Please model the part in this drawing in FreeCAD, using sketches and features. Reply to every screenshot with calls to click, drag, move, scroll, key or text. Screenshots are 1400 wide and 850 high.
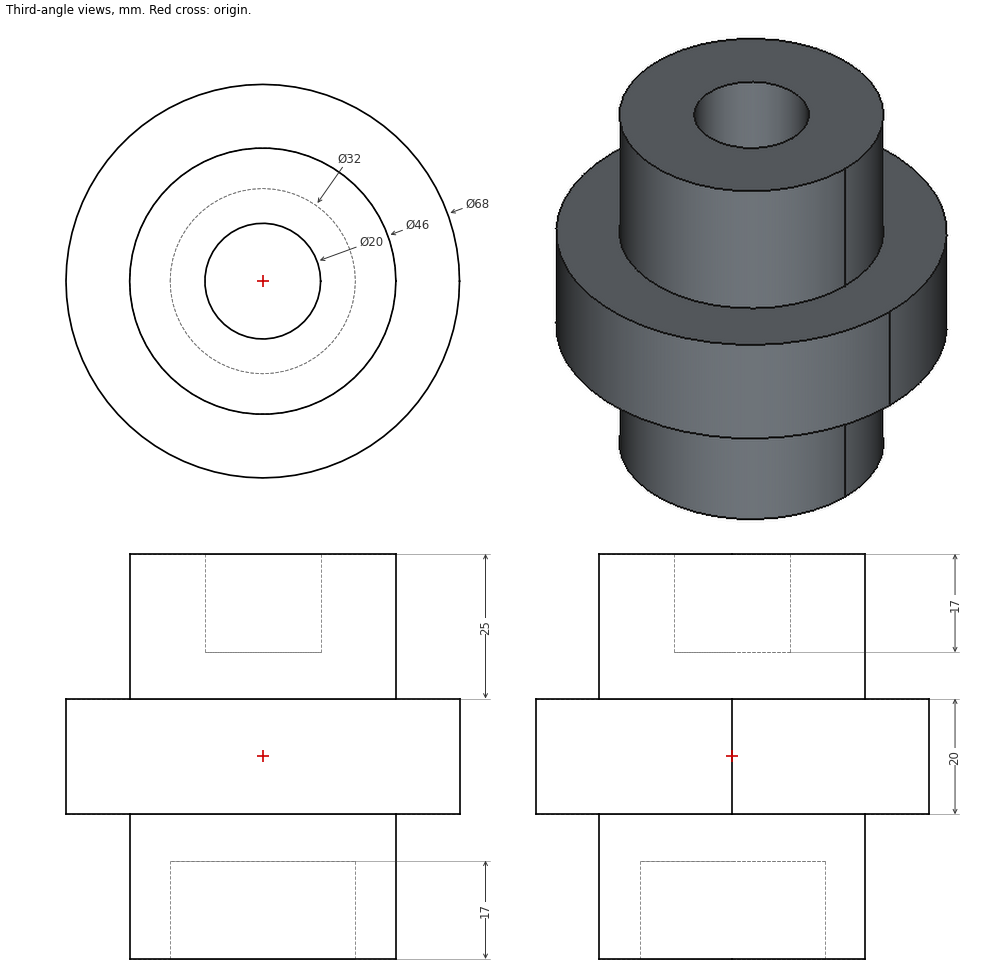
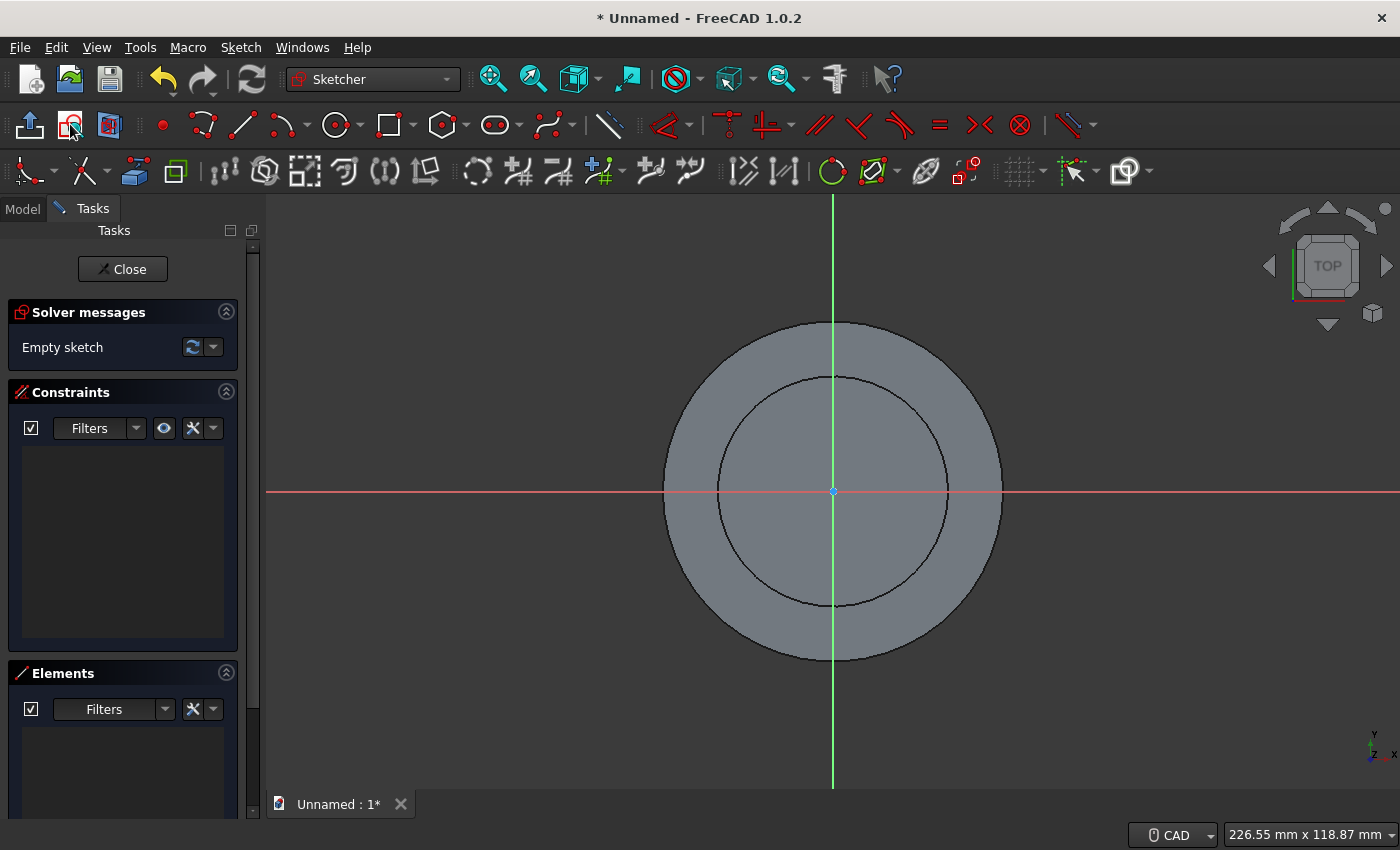
scroll(855, 492, up, 7)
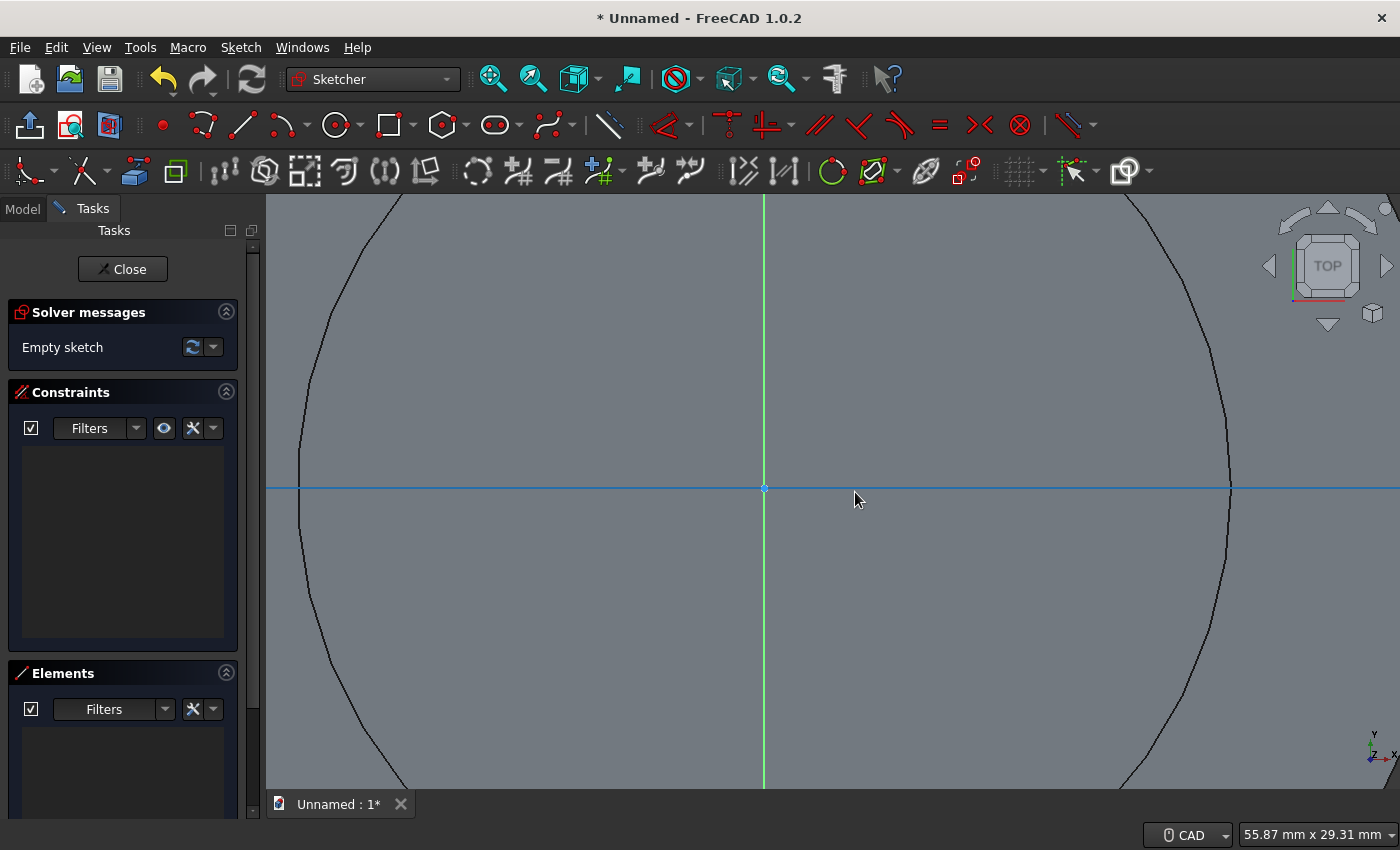
click(336, 126)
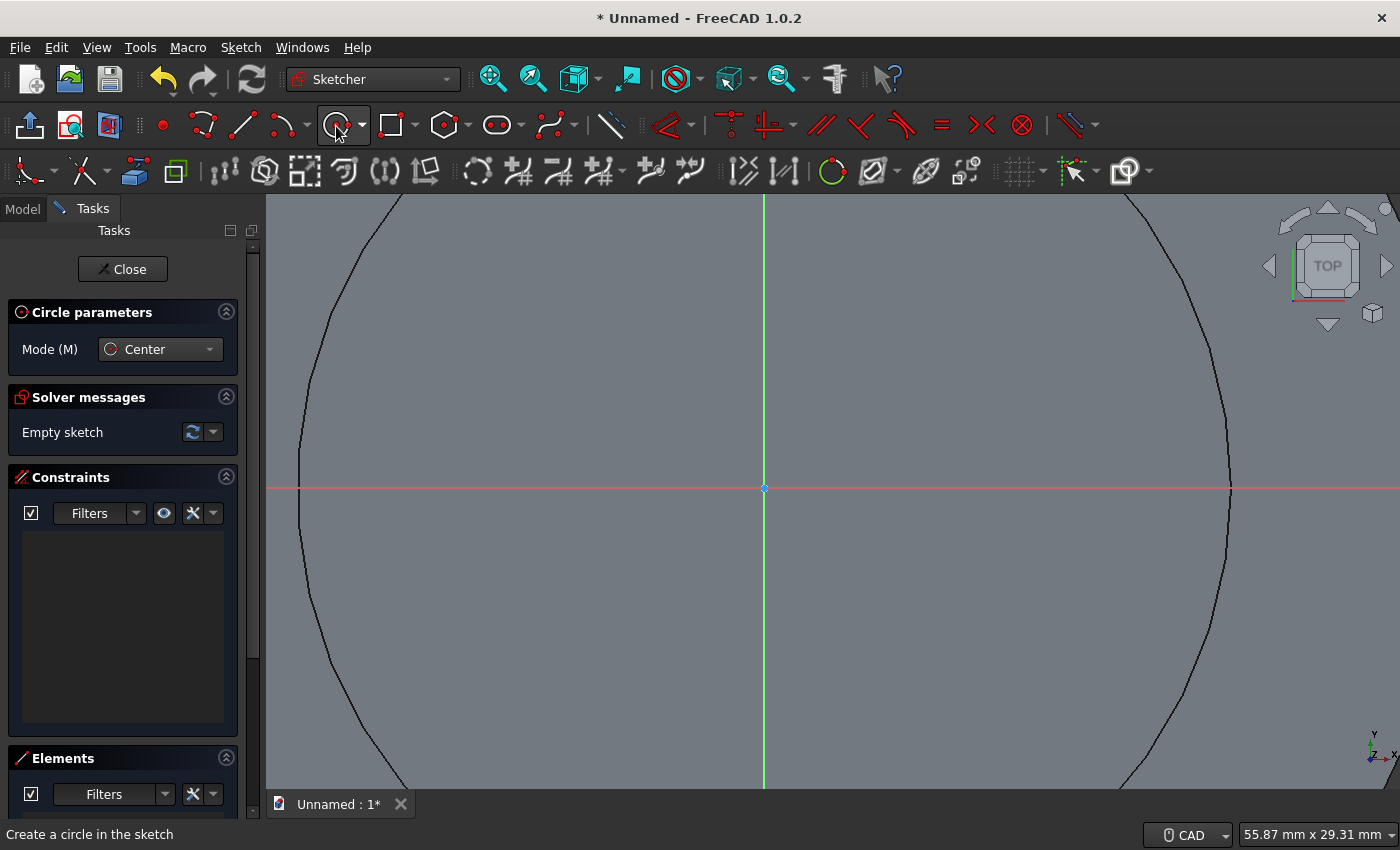
click(764, 488)
move(908, 345)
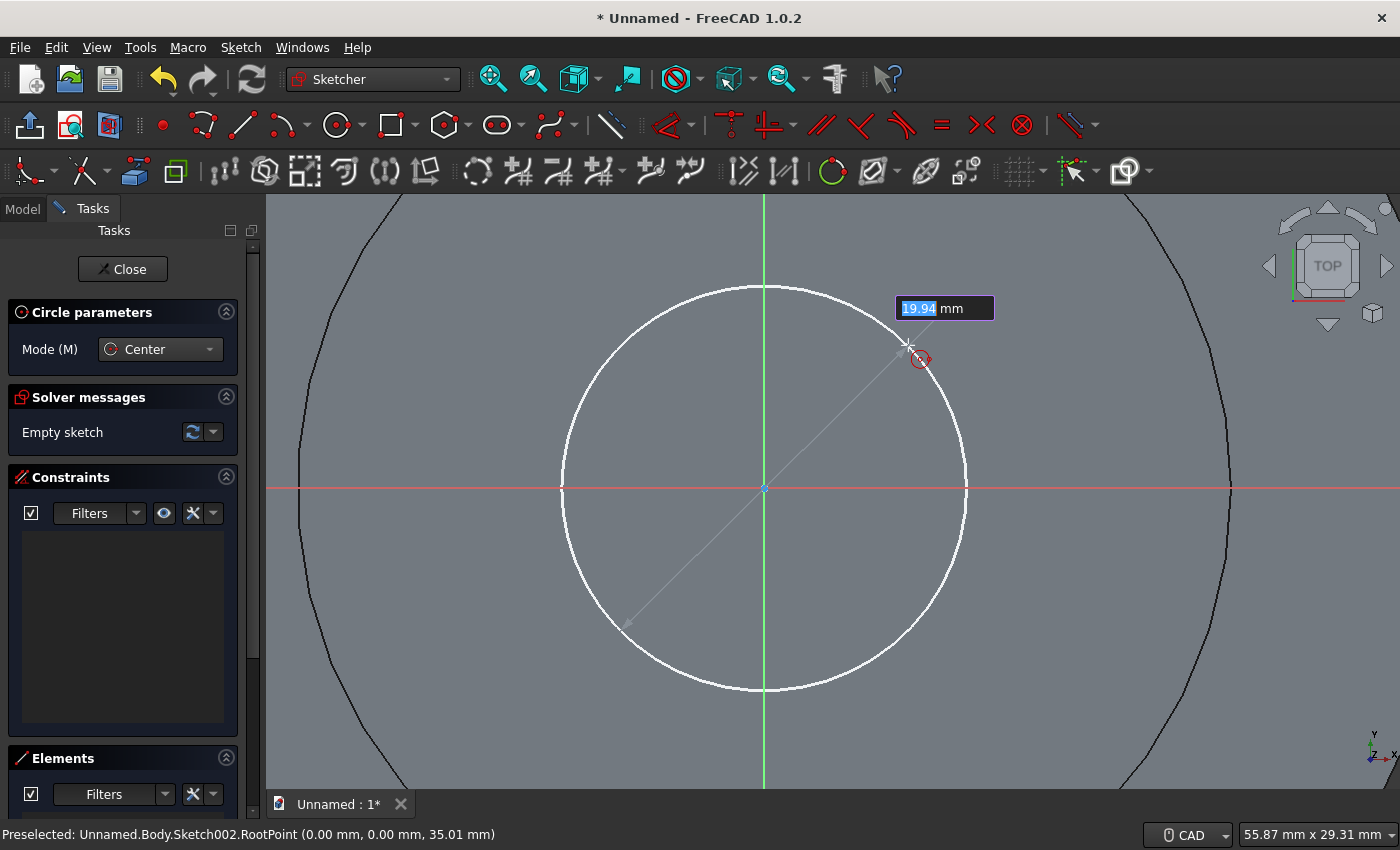
text(20)
key(Return)
key(Escape)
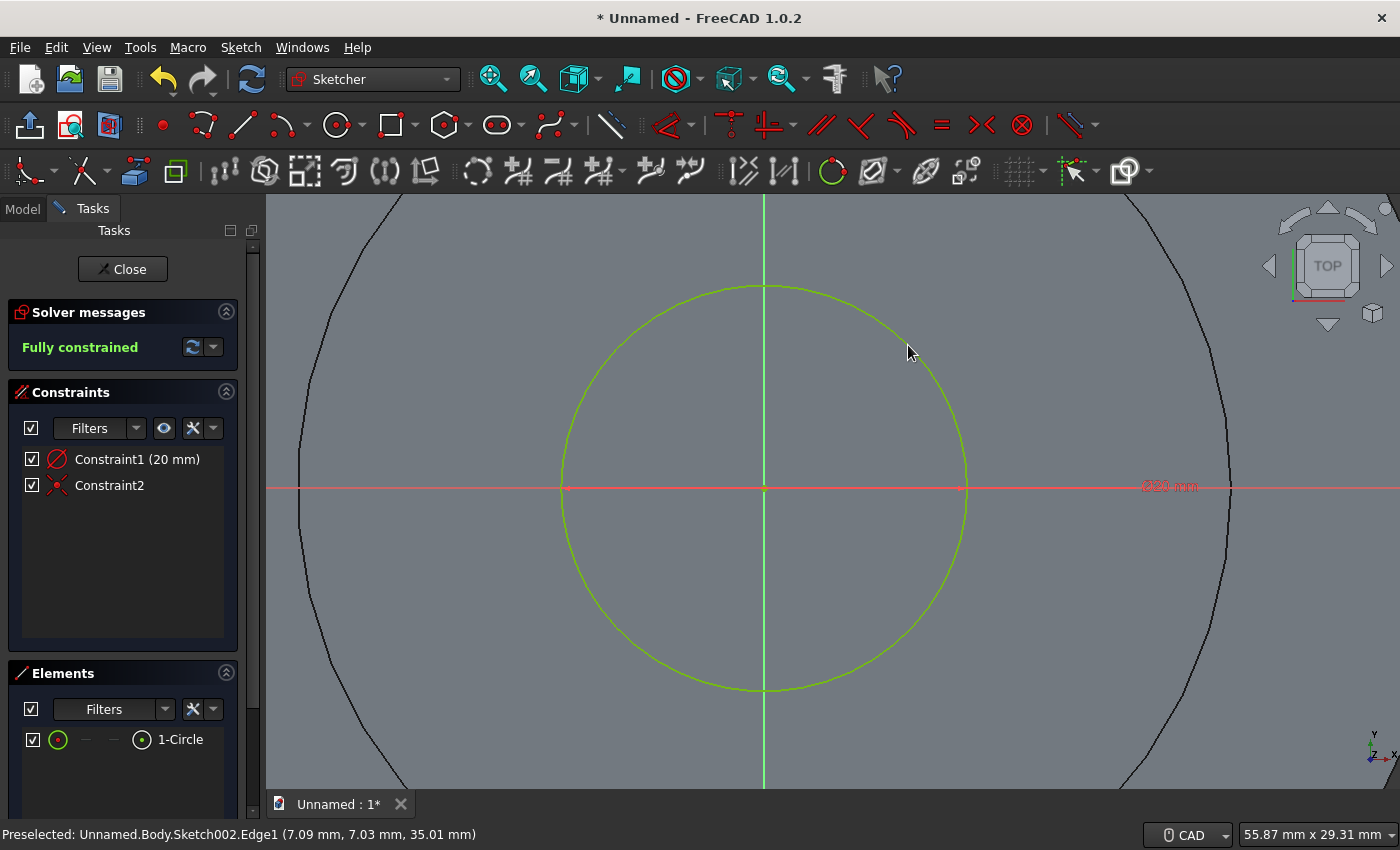
click(123, 269)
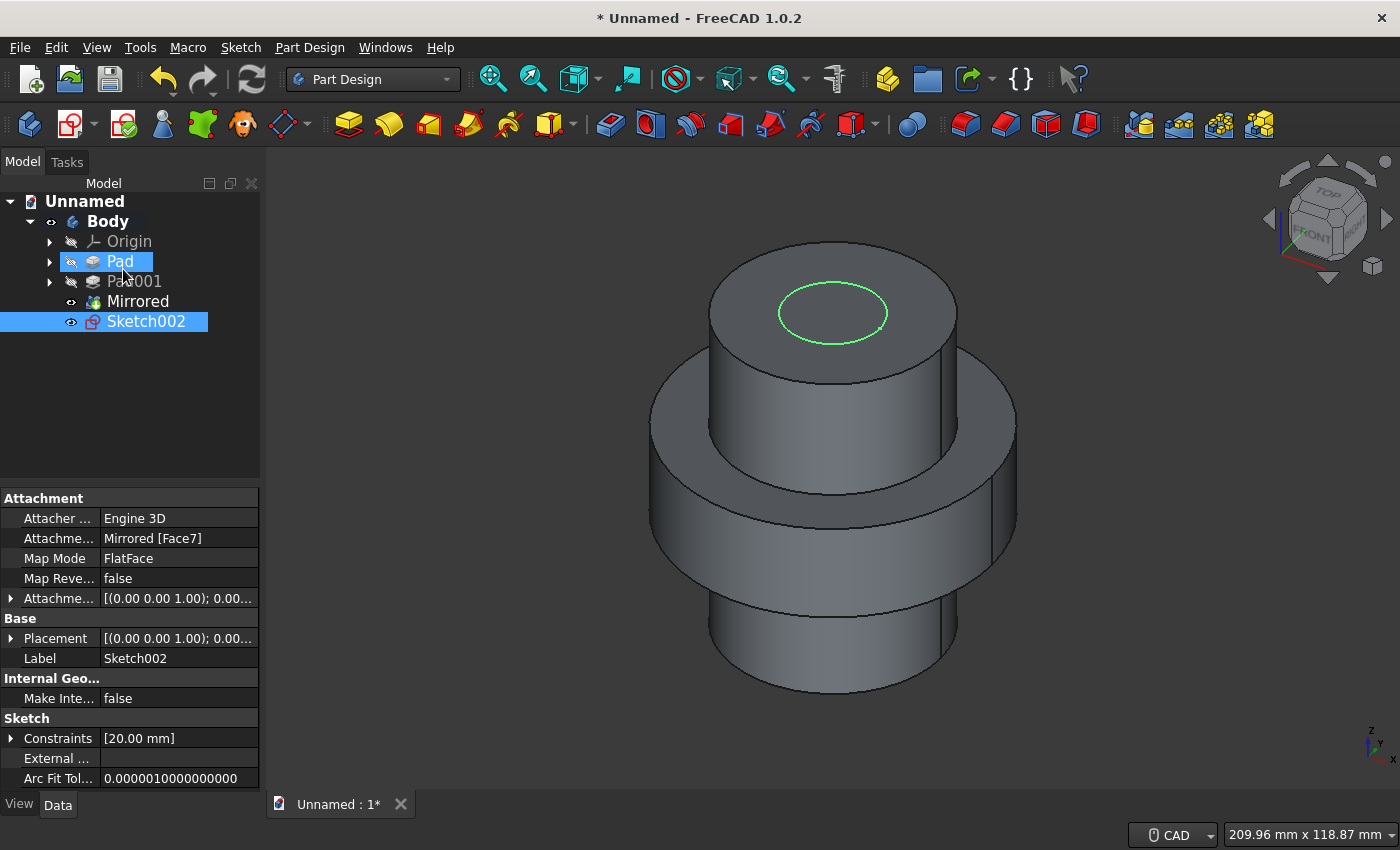
click(612, 124)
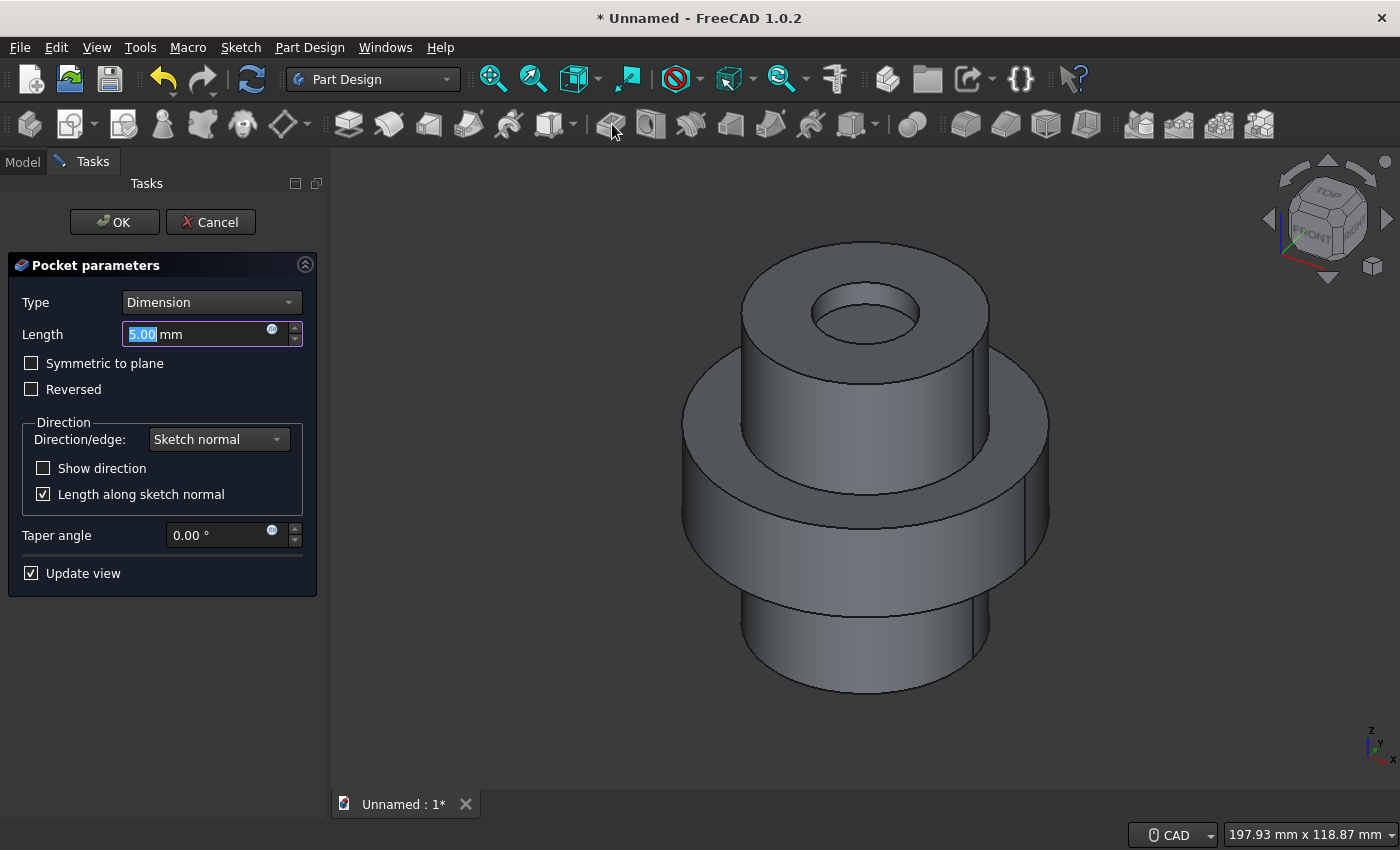
text(17)
key(Tab)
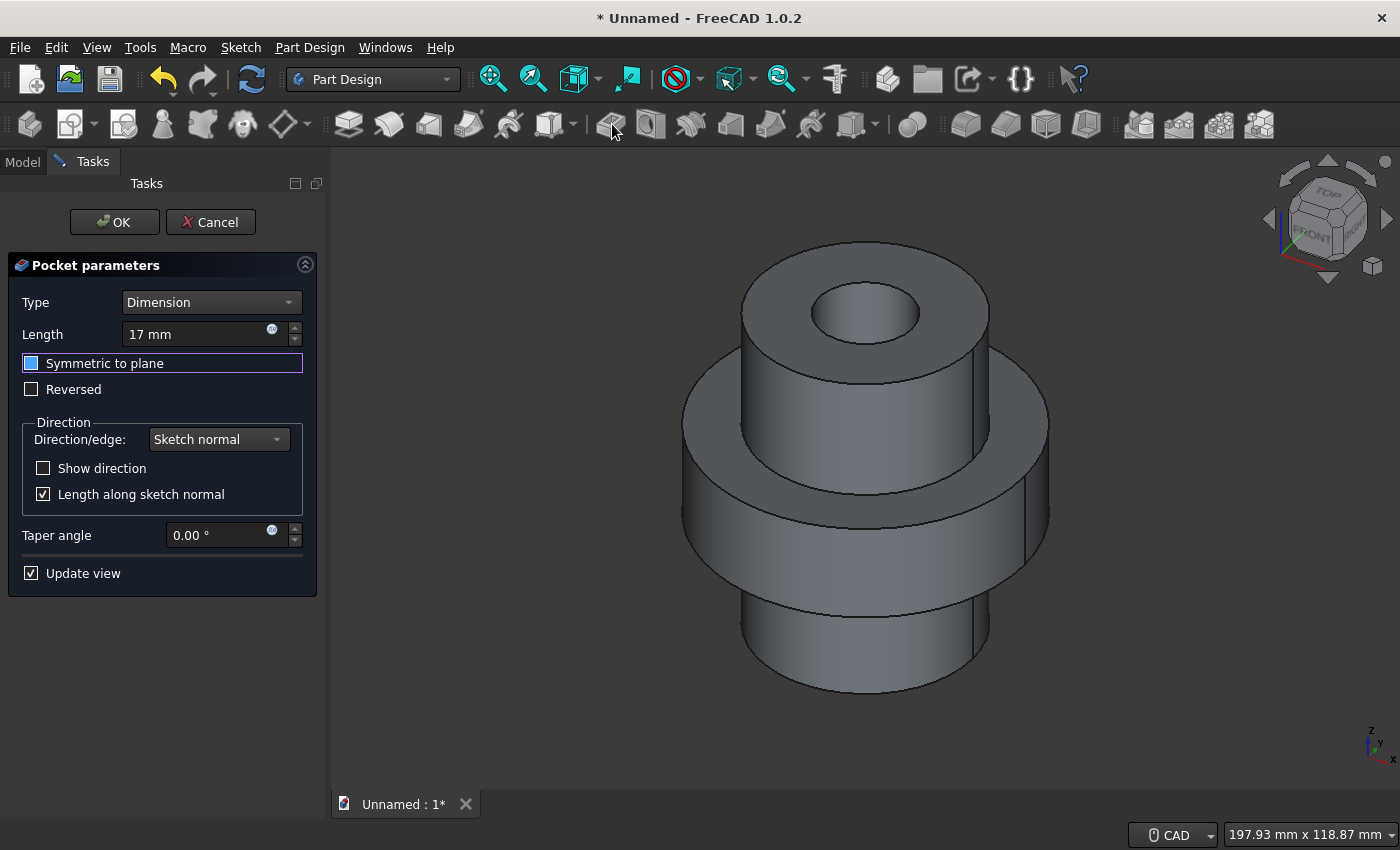
click(115, 222)